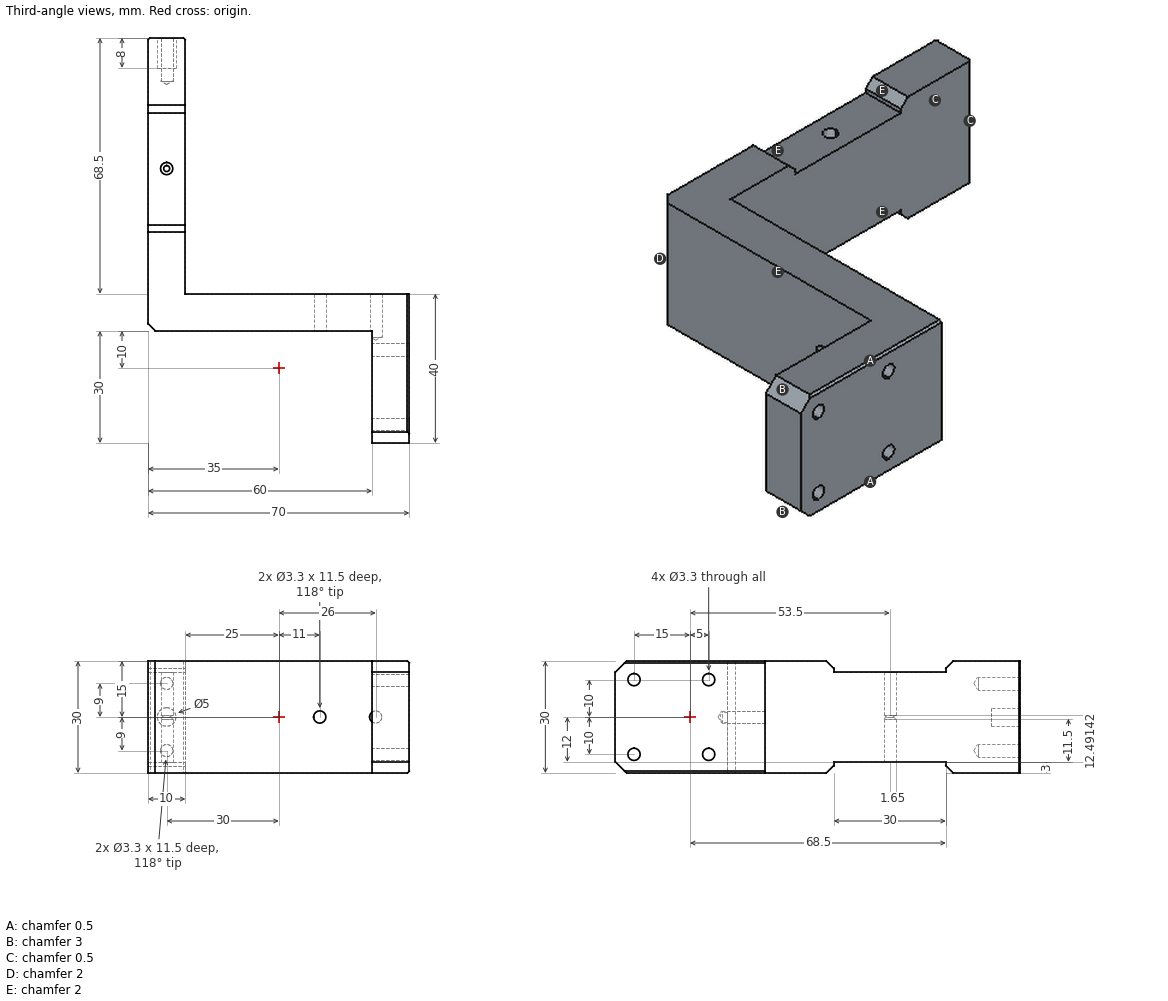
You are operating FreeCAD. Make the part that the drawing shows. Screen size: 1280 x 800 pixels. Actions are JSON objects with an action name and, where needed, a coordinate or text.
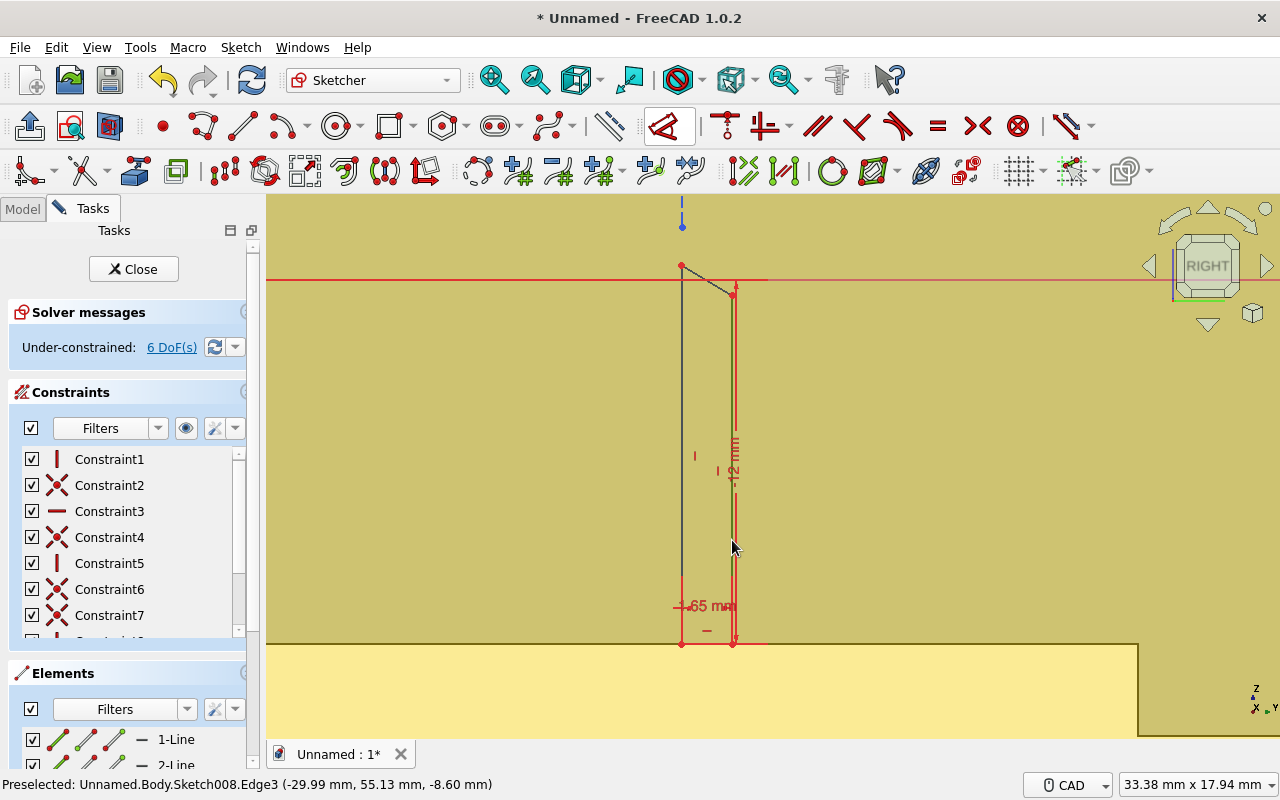
{"action": "left_click", "coordinate": [690, 126]}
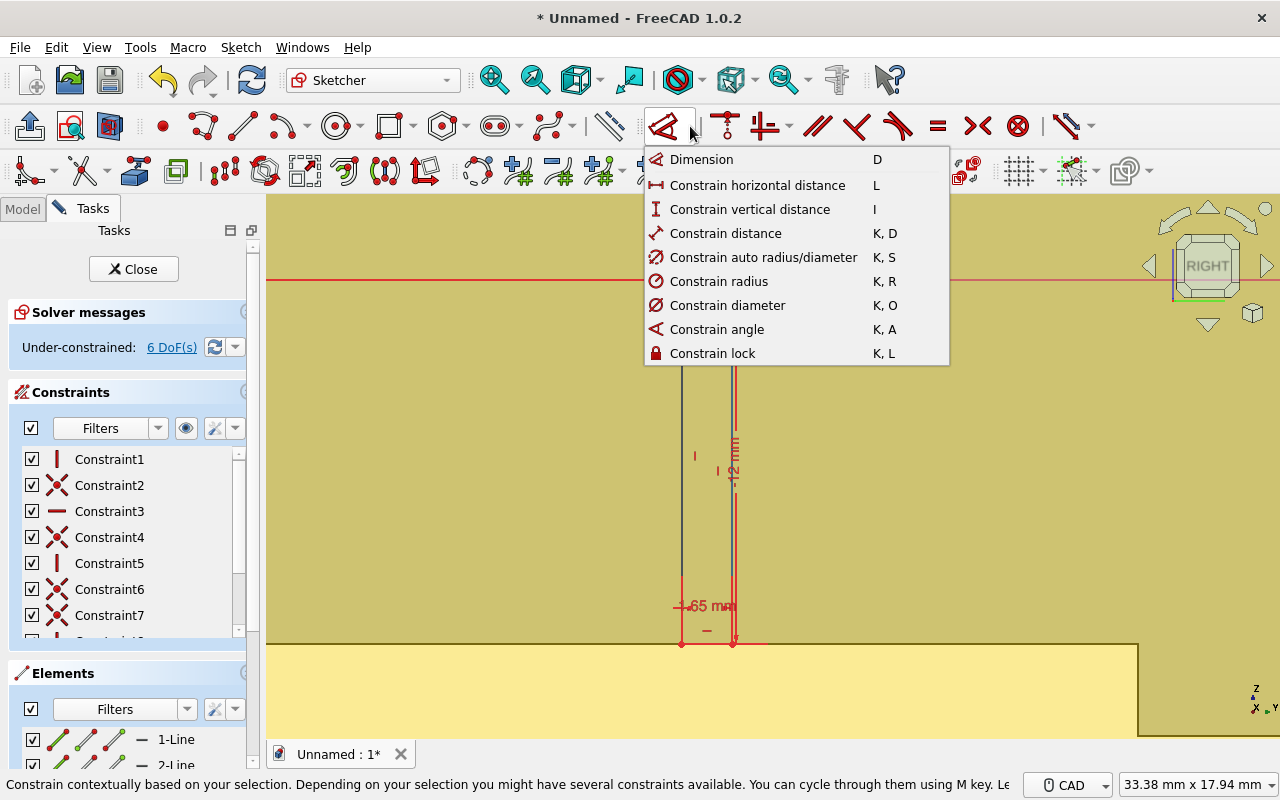
{"action": "left_click", "coordinate": [797, 209]}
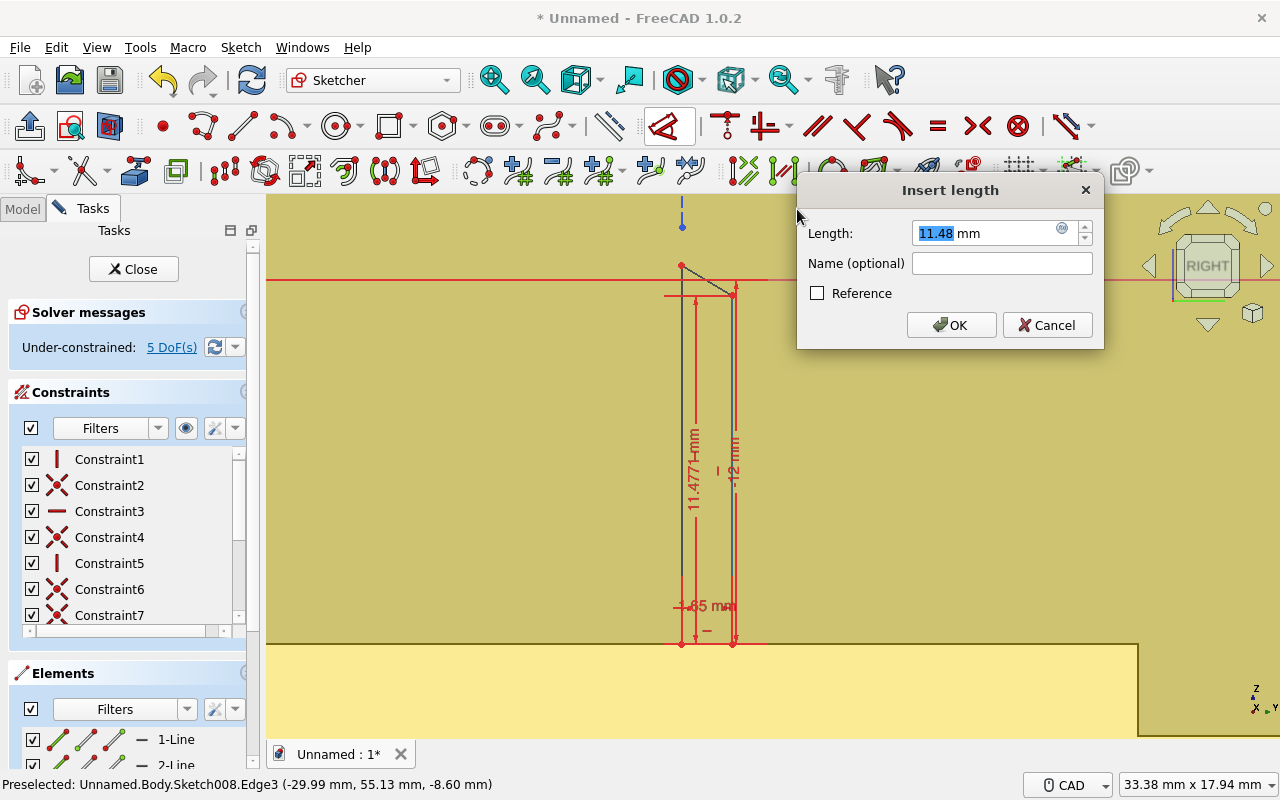
{"action": "type", "text": "11.5"}
{"action": "key", "text": "Return"}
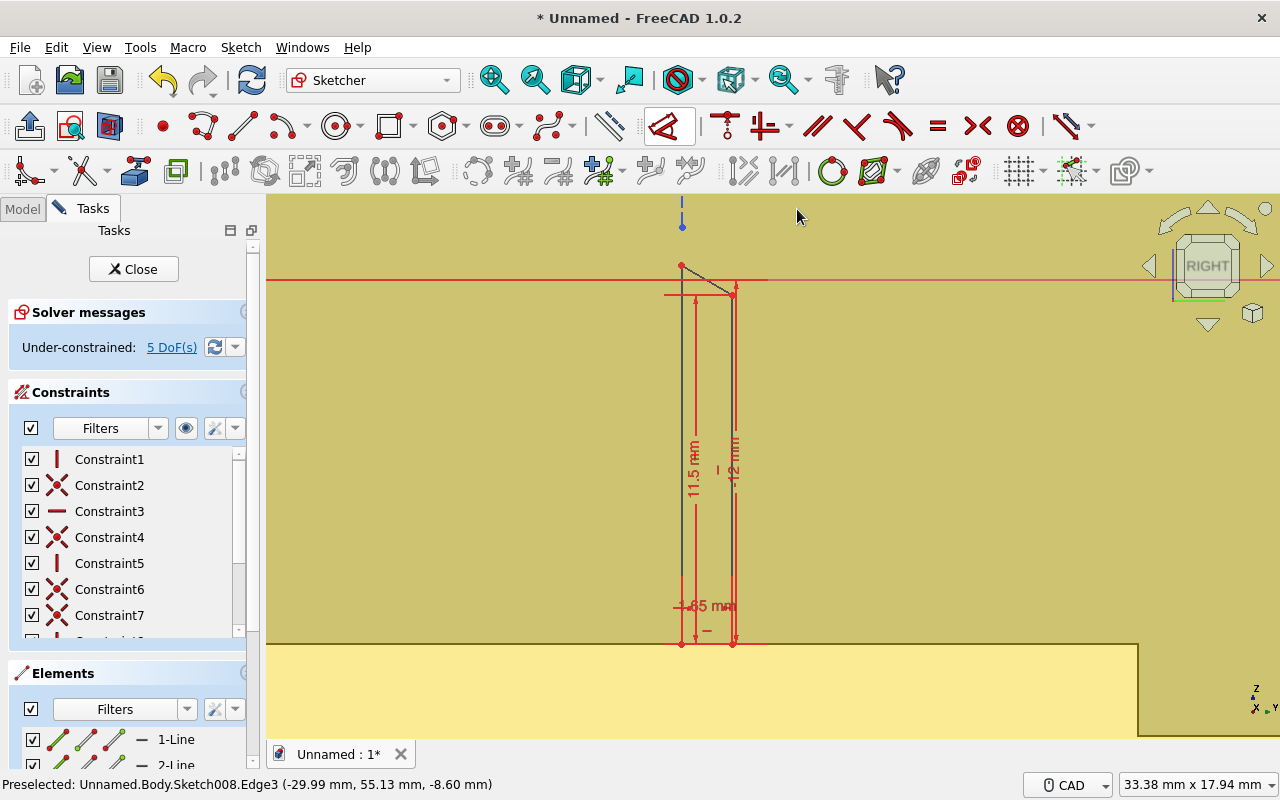
{"action": "left_click", "coordinate": [682, 266]}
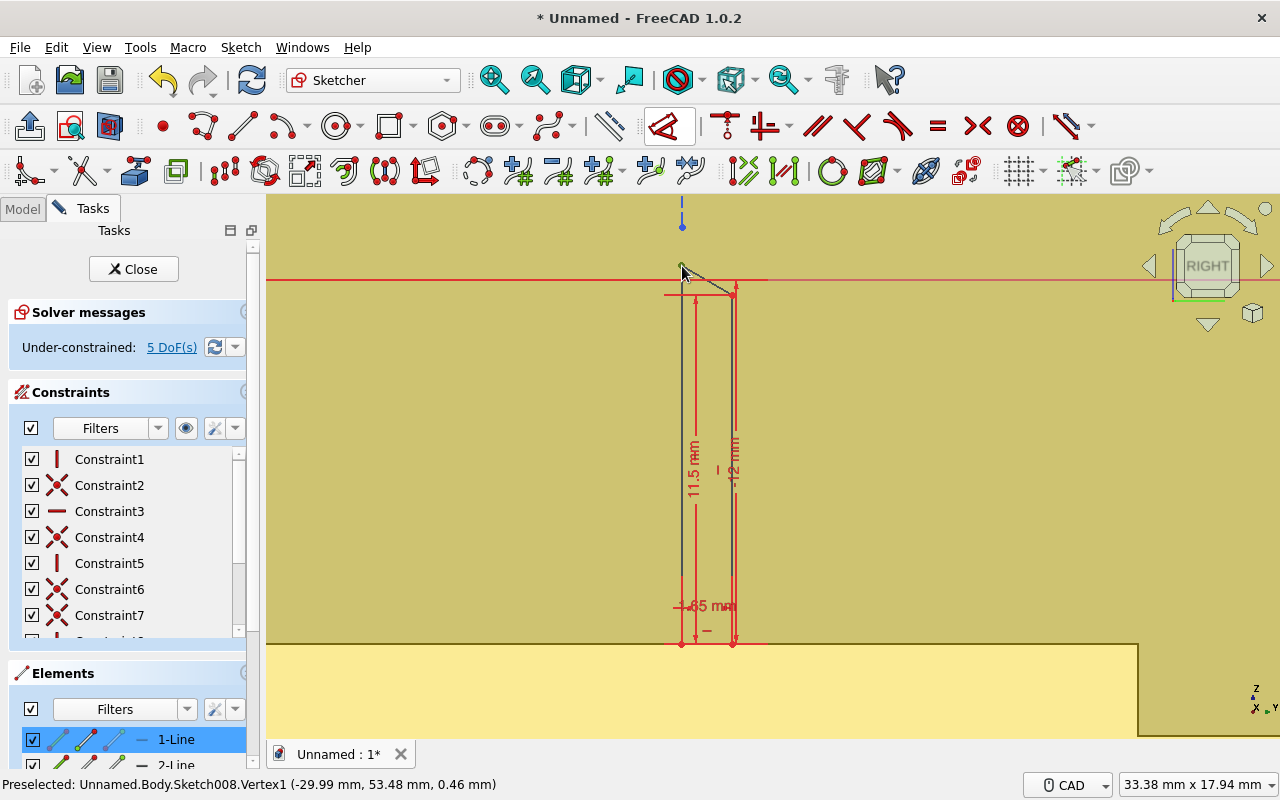
{"action": "key", "text": "l"}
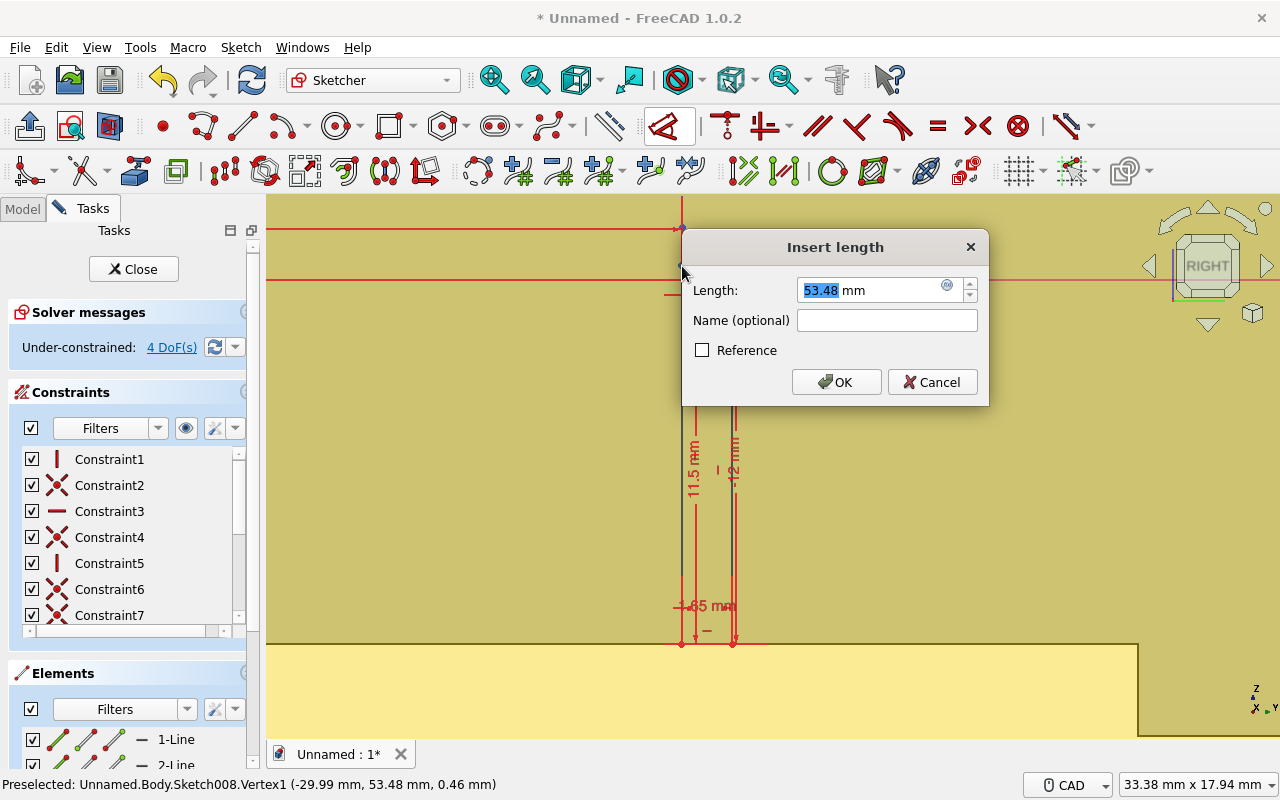
{"action": "type", "text": "53.5"}
{"action": "key", "text": "Return"}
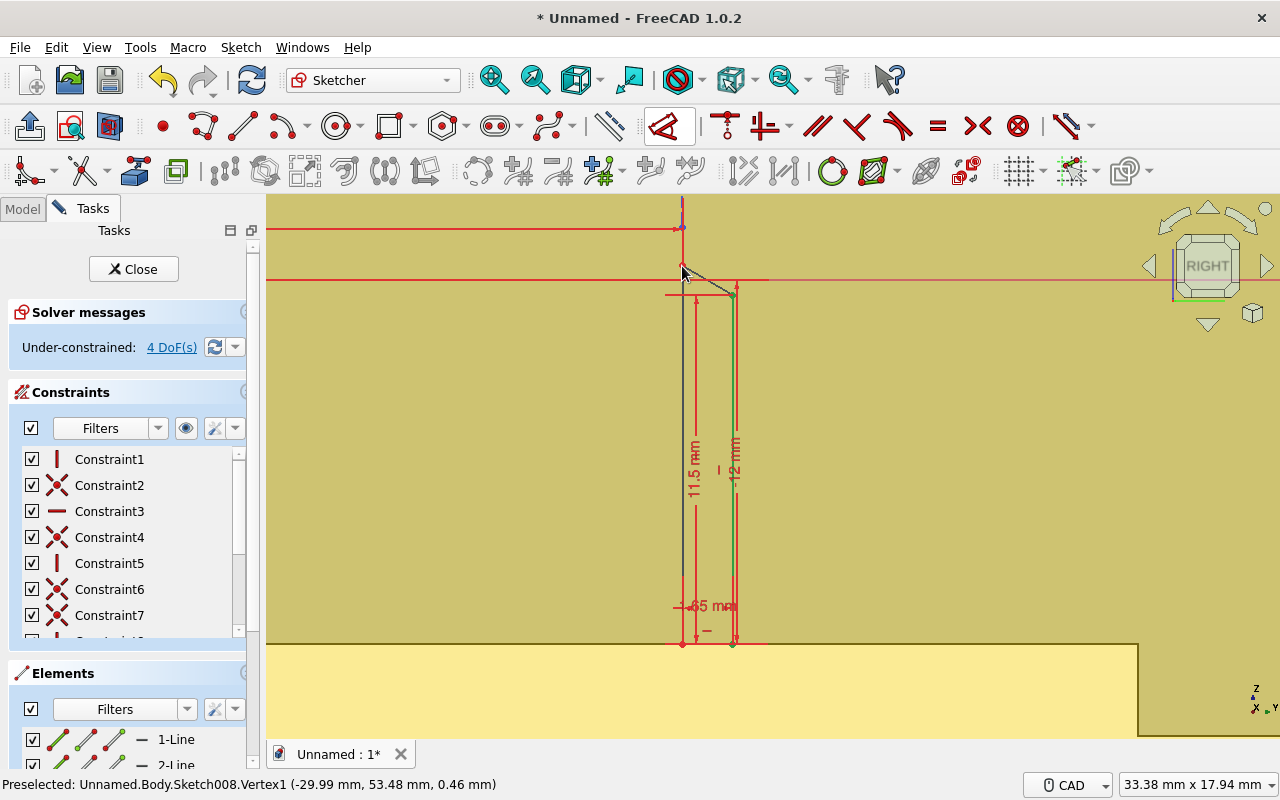
{"action": "left_click", "coordinate": [682, 228]}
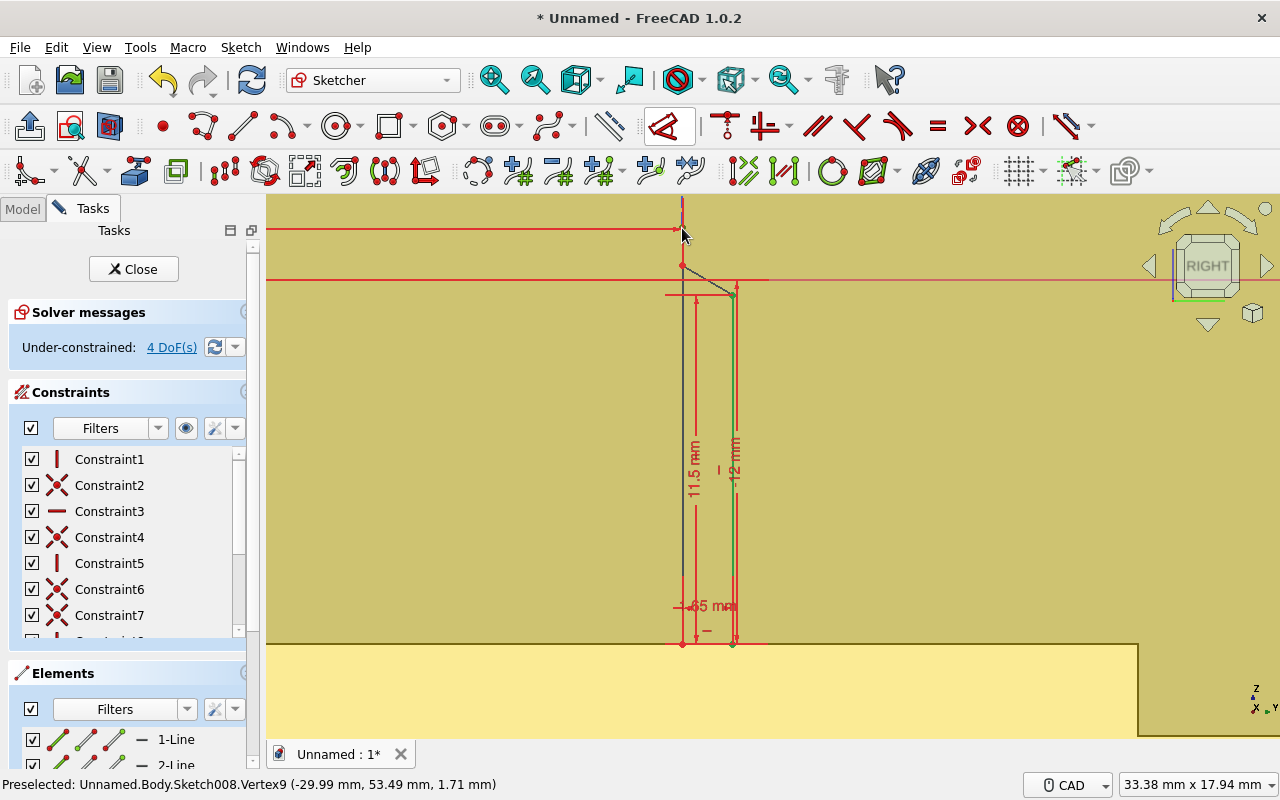
{"action": "left_click", "coordinate": [690, 126]}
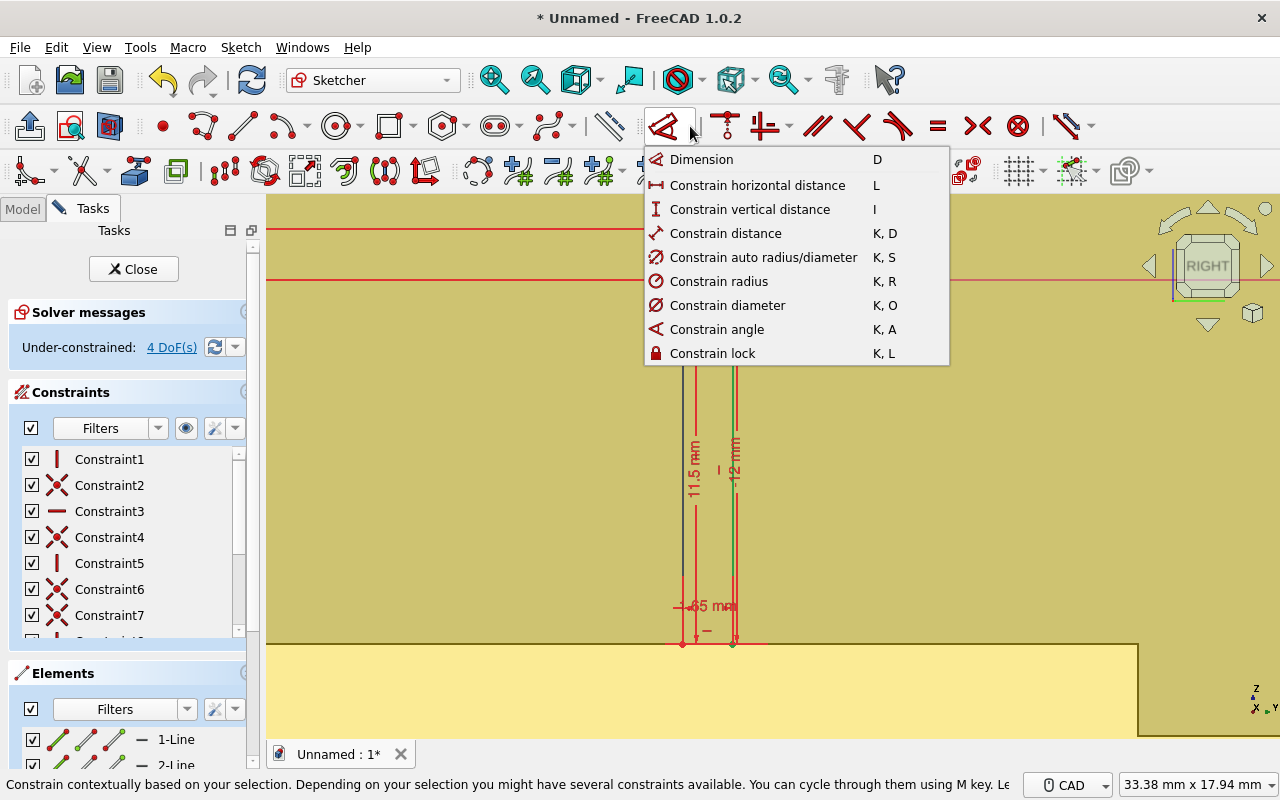
{"action": "left_click", "coordinate": [797, 185]}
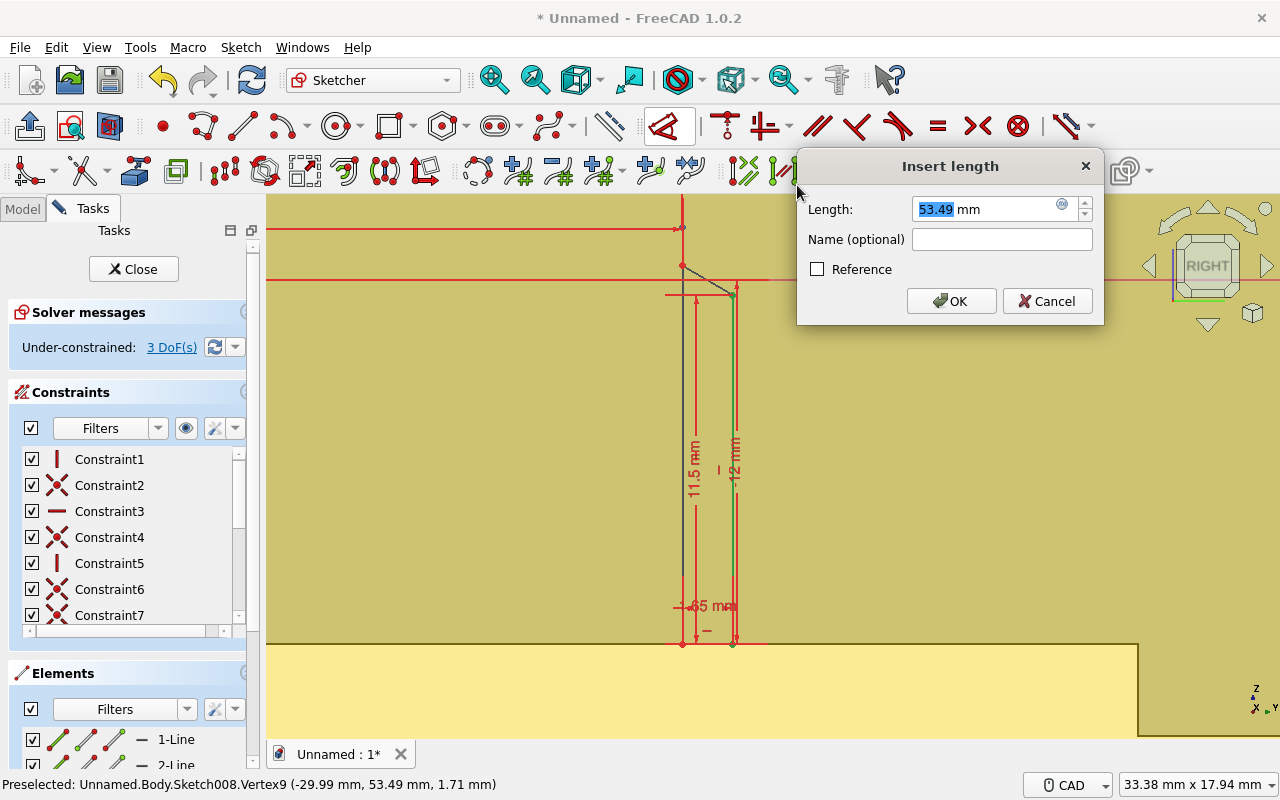
{"action": "type", "text": "53.5"}
{"action": "key", "text": "Return"}